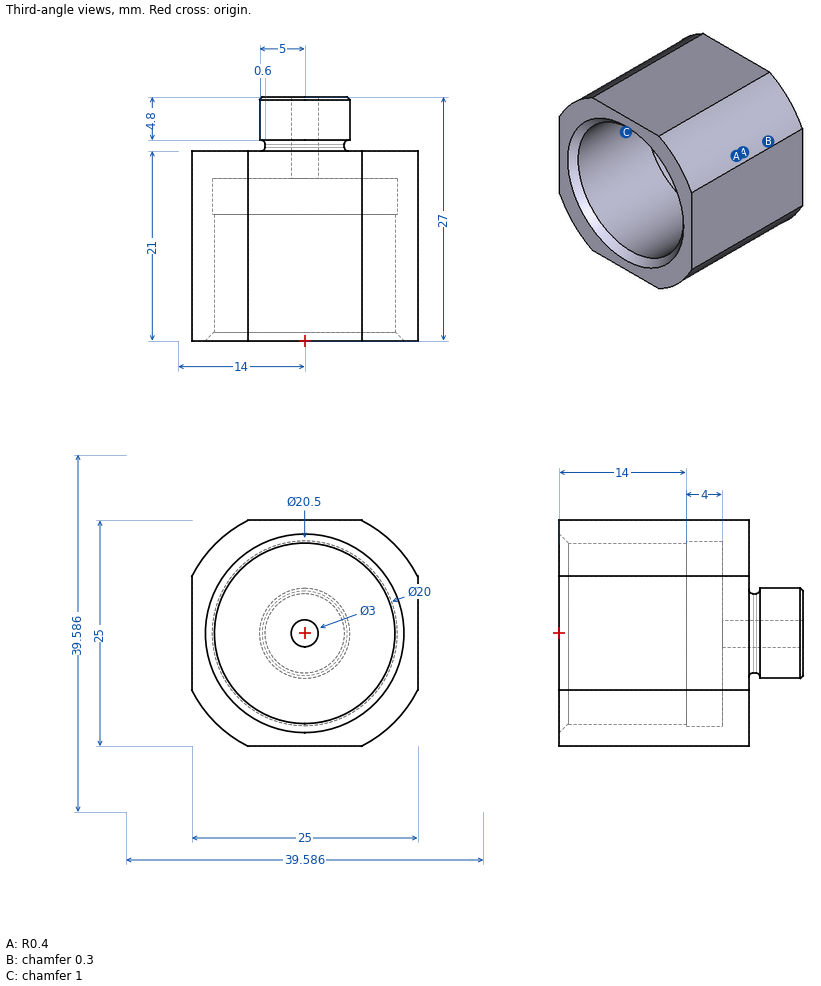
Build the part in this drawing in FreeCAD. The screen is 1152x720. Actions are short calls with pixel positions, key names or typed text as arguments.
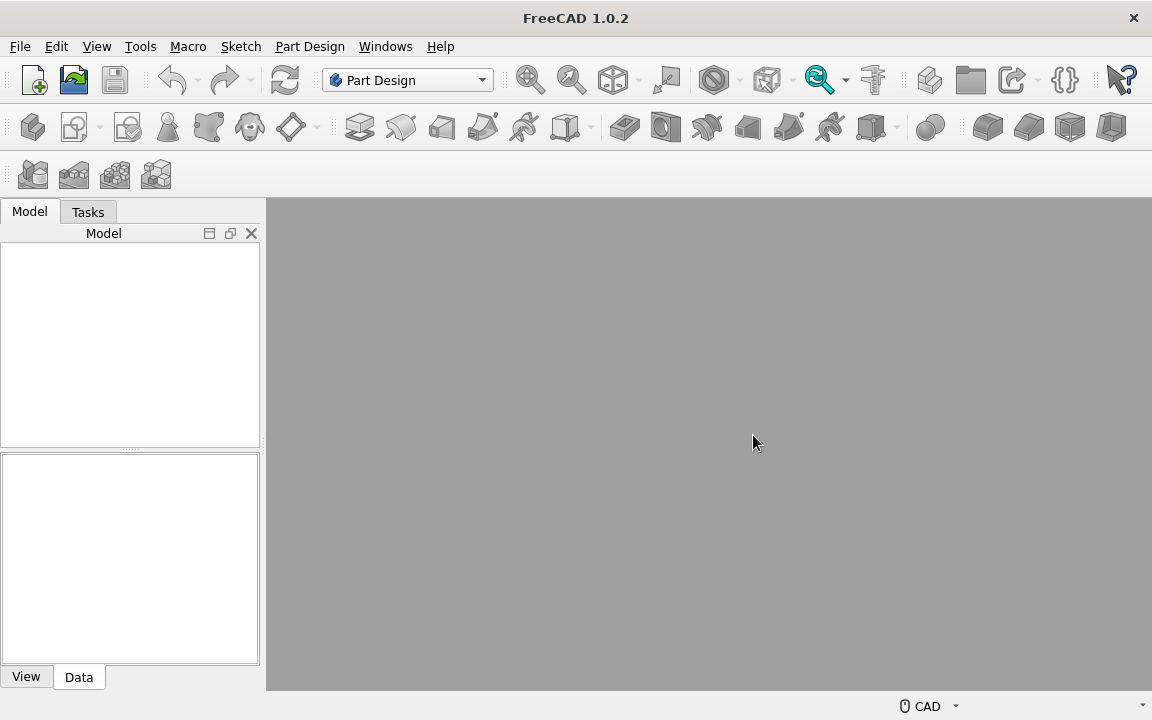
click(33, 80)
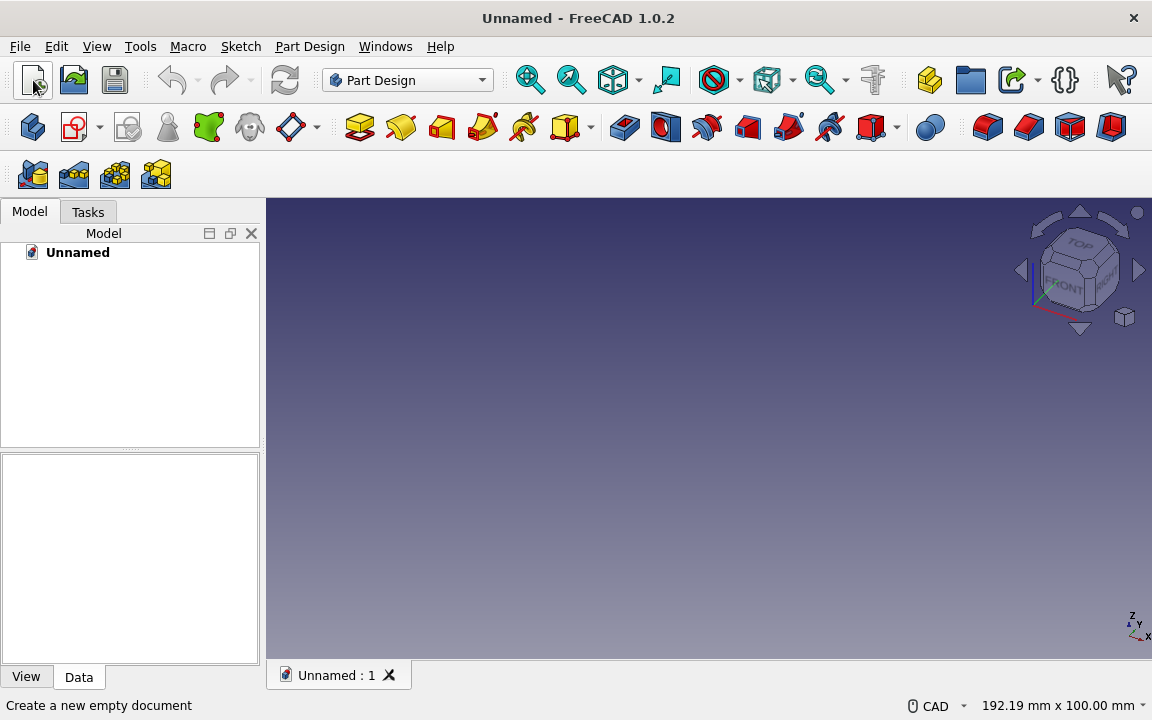
click(74, 128)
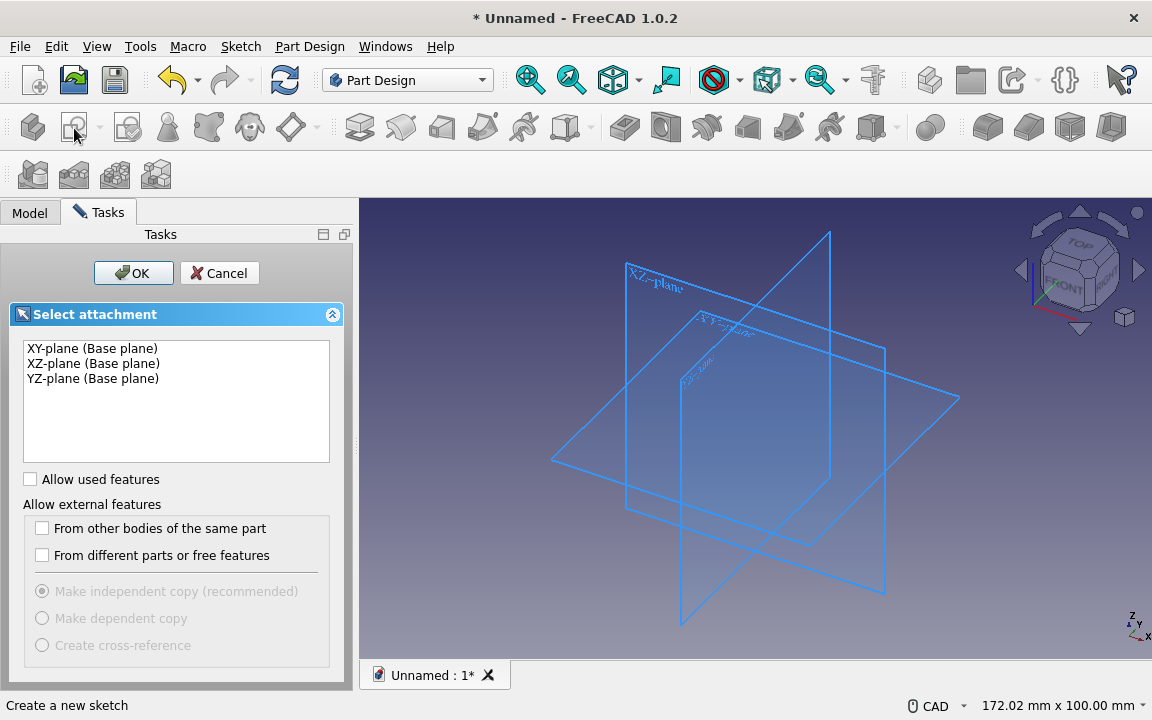
click(84, 348)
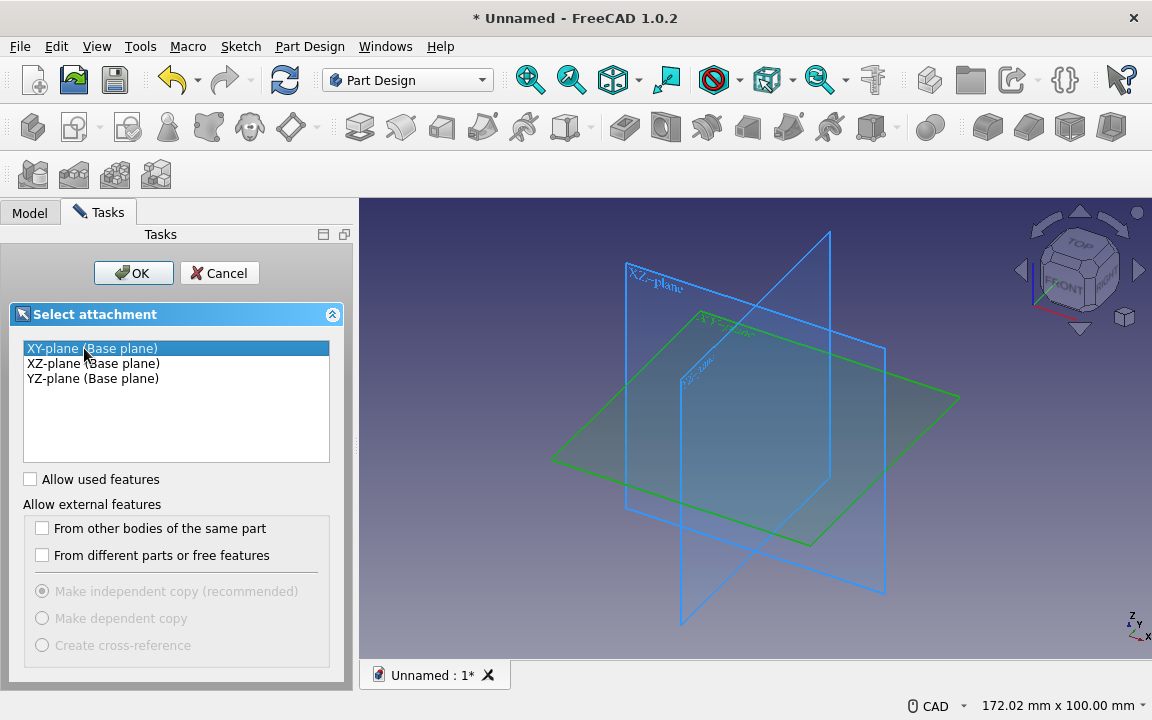
click(134, 273)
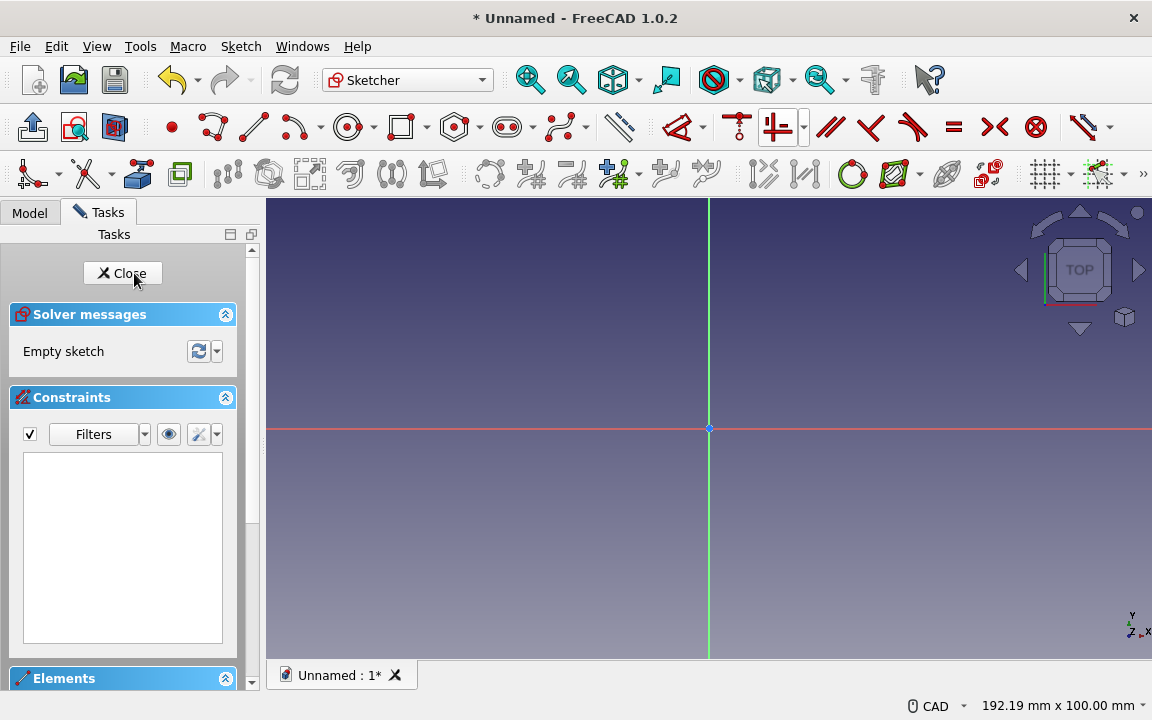
scroll(706, 315, up, 4)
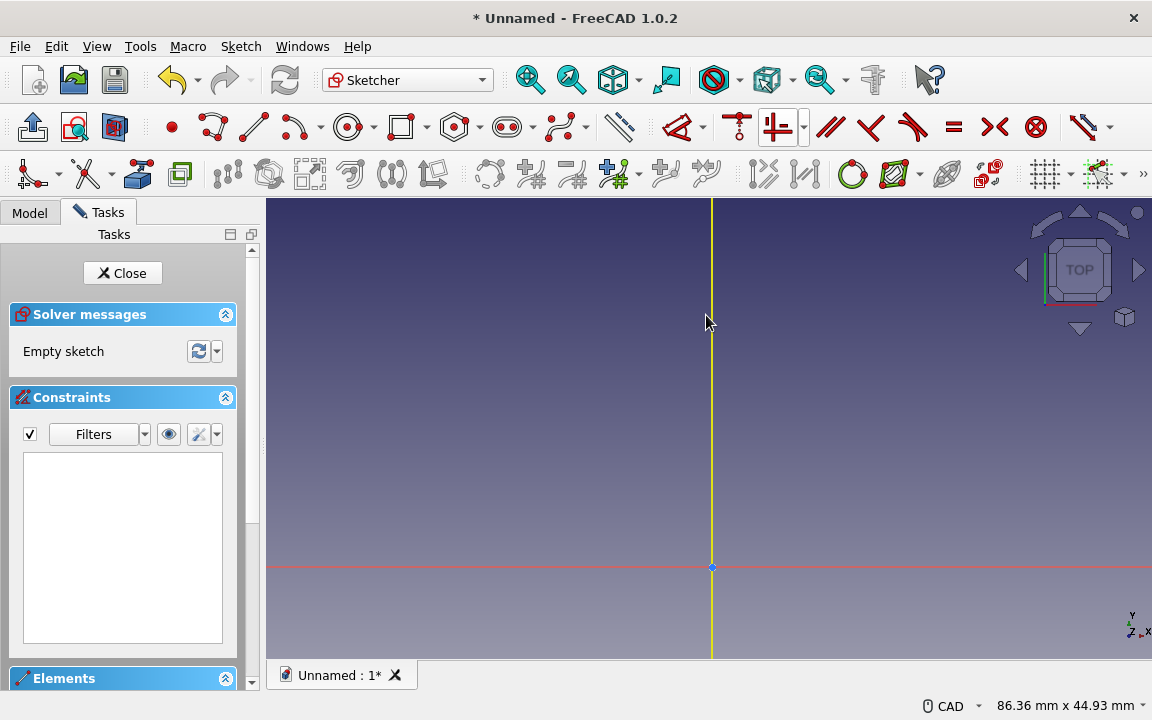
click(213, 128)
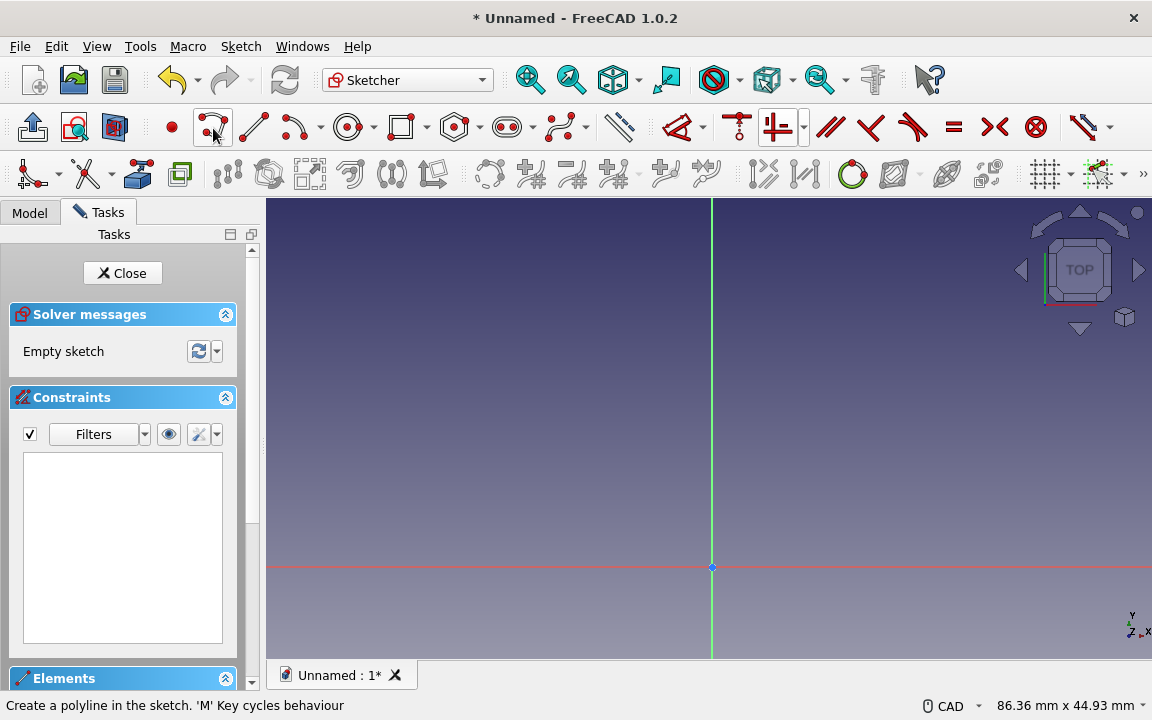
click(712, 567)
click(703, 290)
click(661, 290)
click(661, 340)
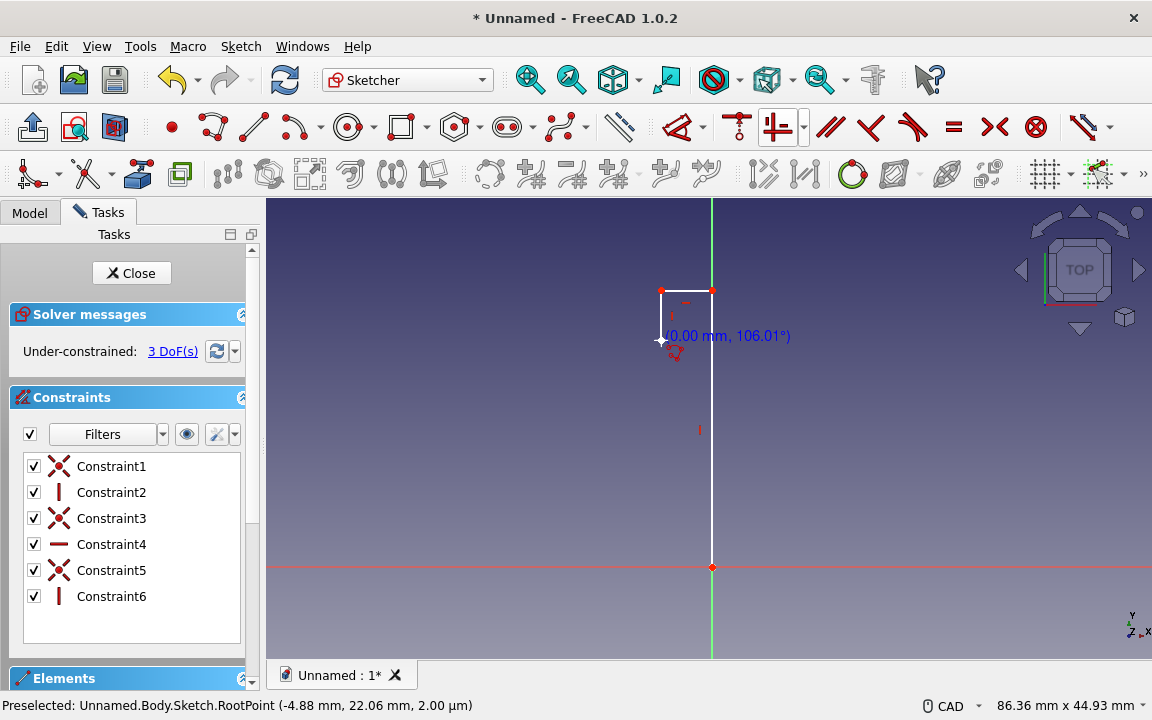
scroll(667, 340, up, 5)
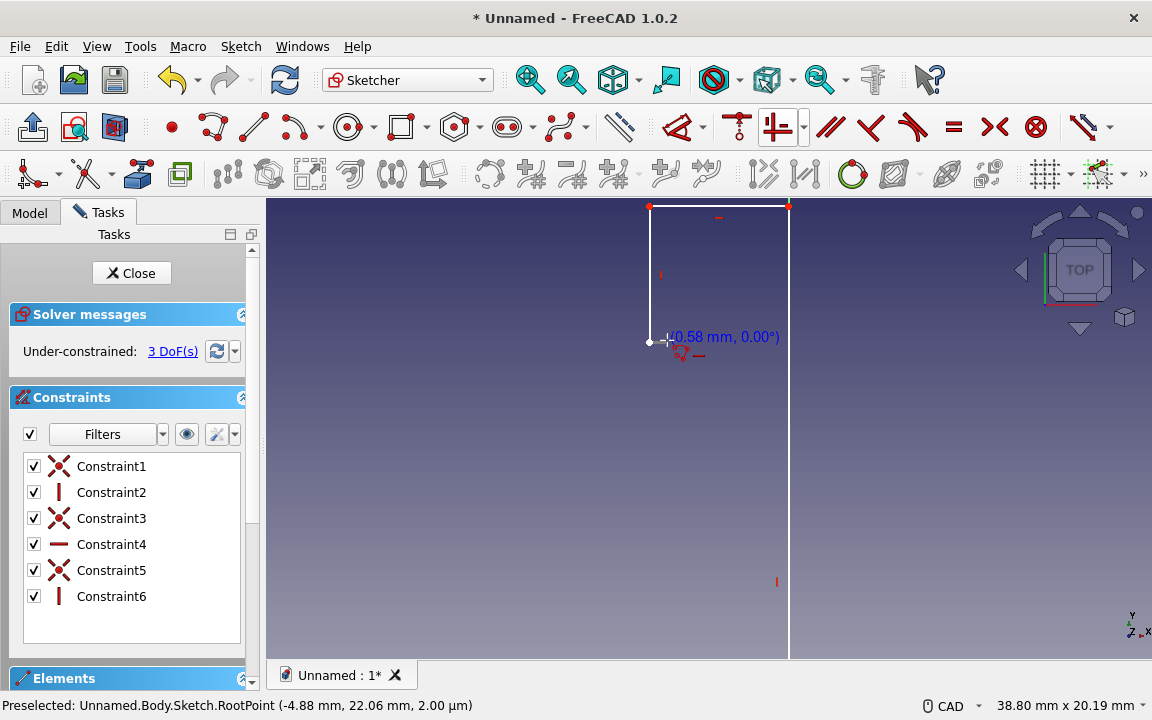
click(666, 339)
click(666, 372)
click(398, 372)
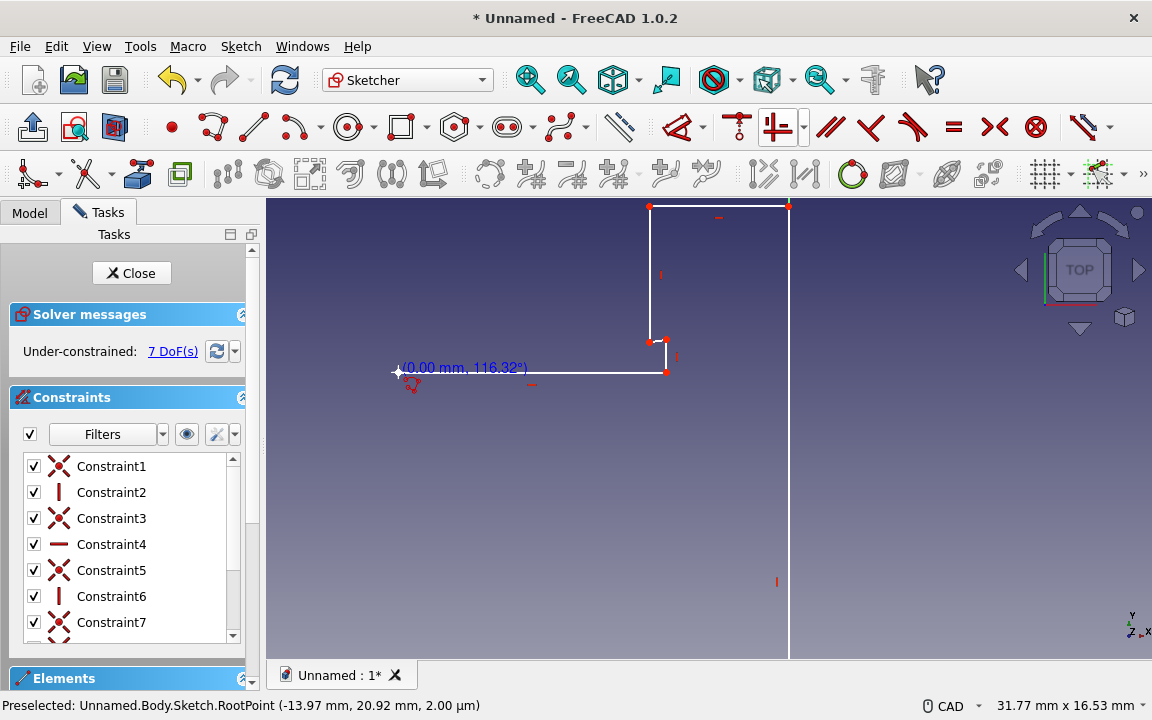
scroll(668, 340, down, 5)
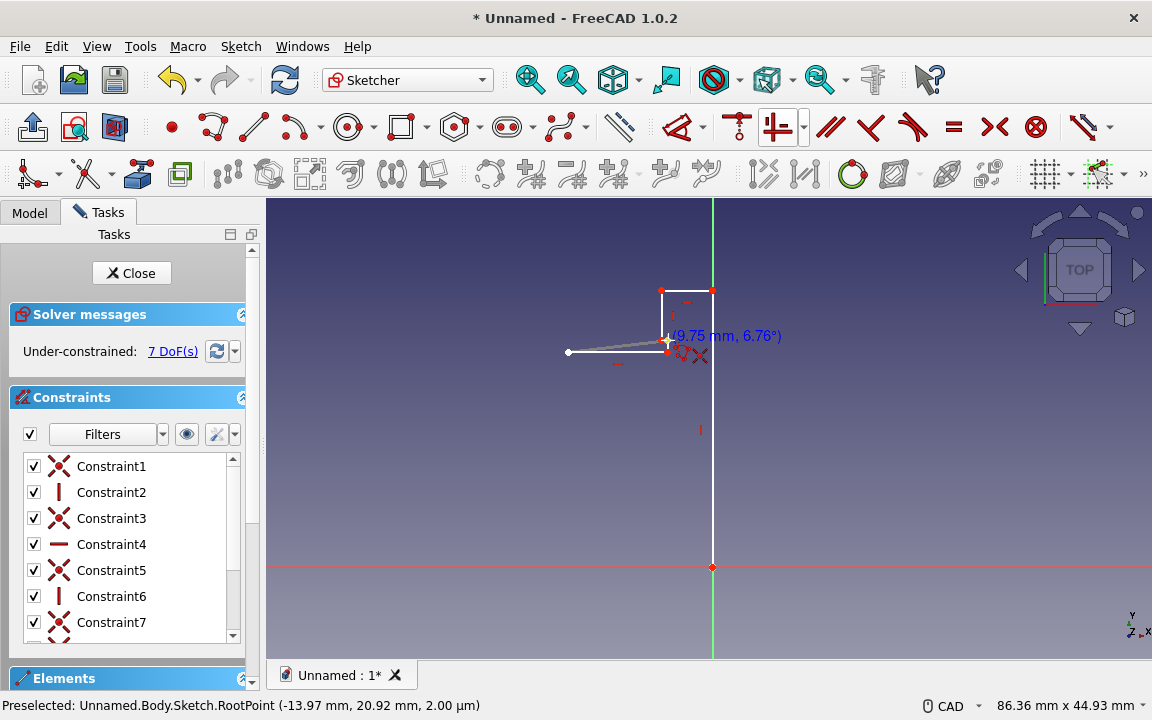
click(569, 558)
click(713, 567)
key(Escape)
key(Escape)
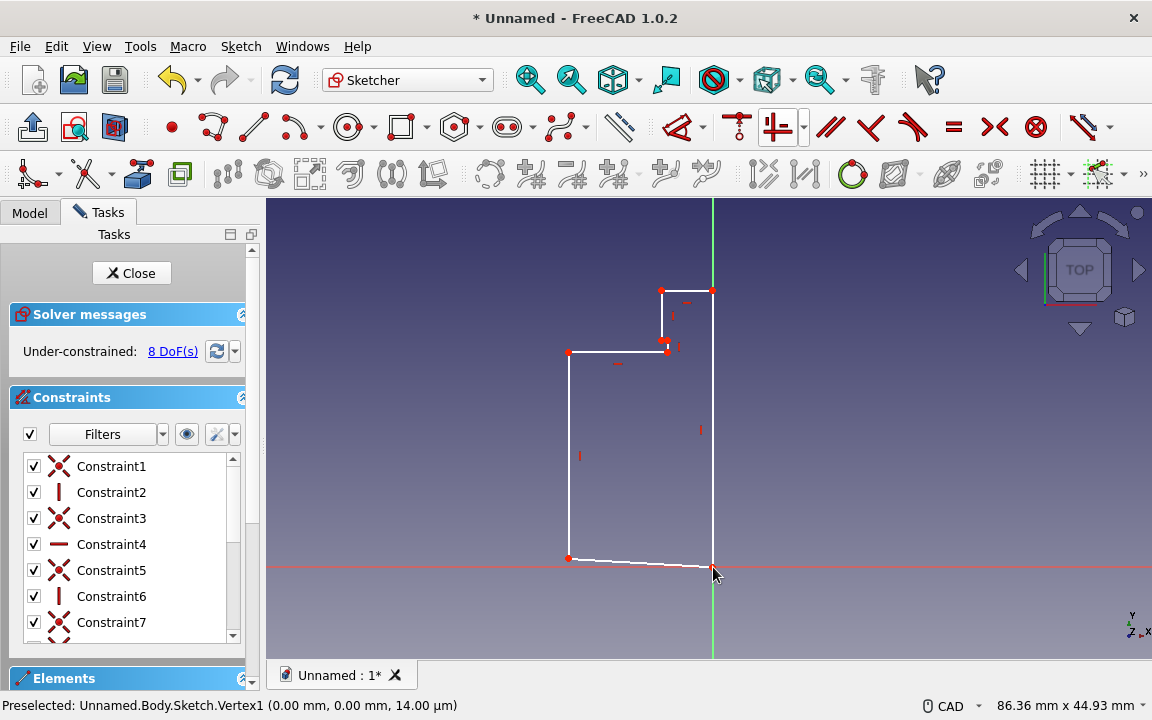
scroll(665, 341, up, 8)